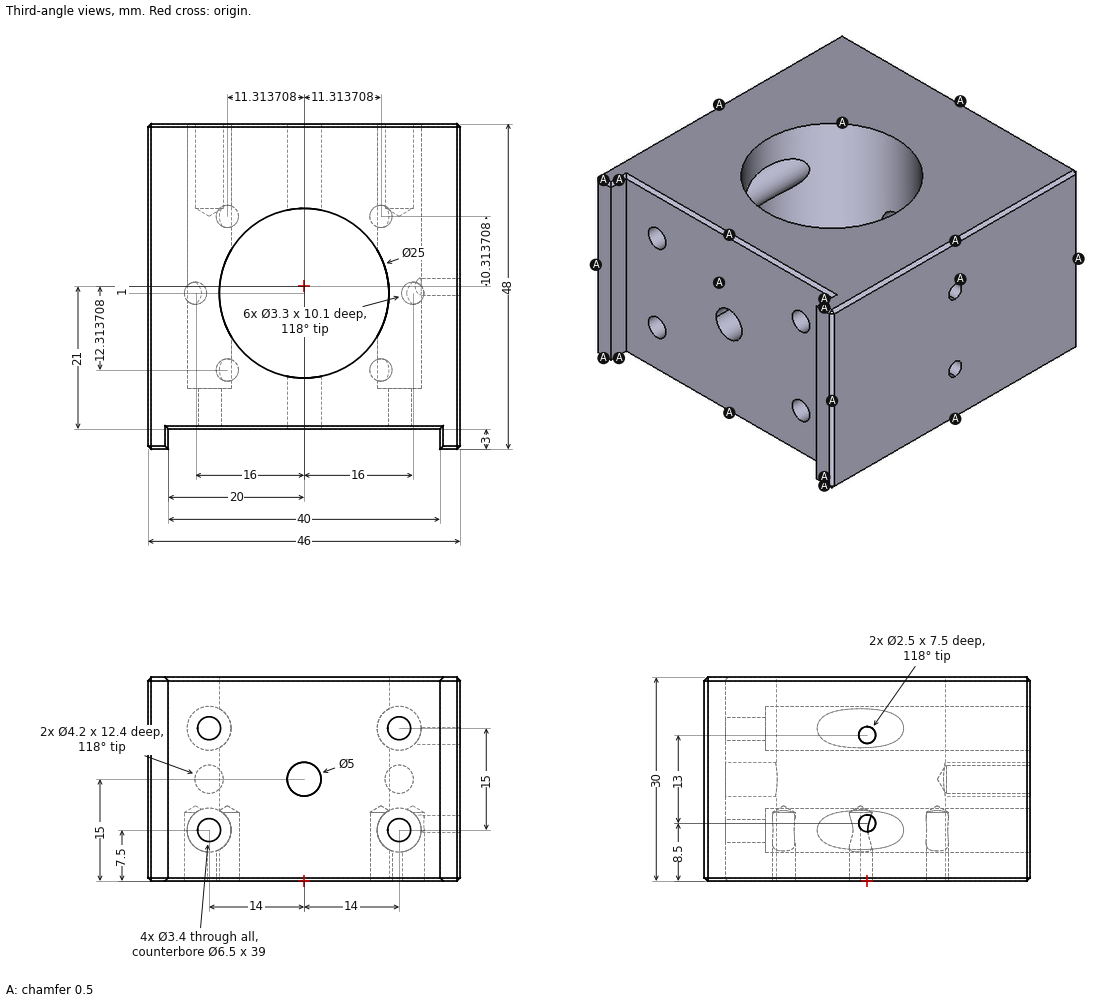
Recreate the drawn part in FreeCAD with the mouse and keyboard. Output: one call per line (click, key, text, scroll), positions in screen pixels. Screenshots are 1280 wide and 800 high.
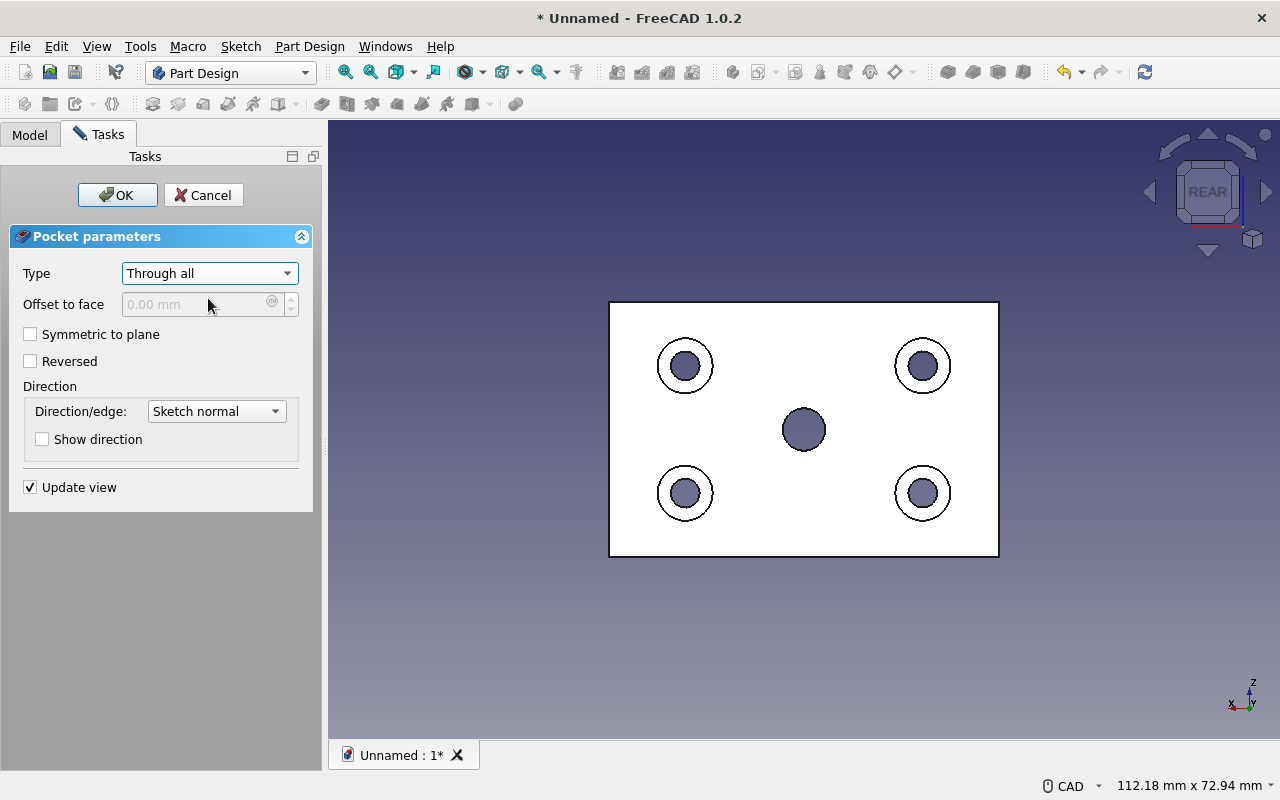
click(118, 195)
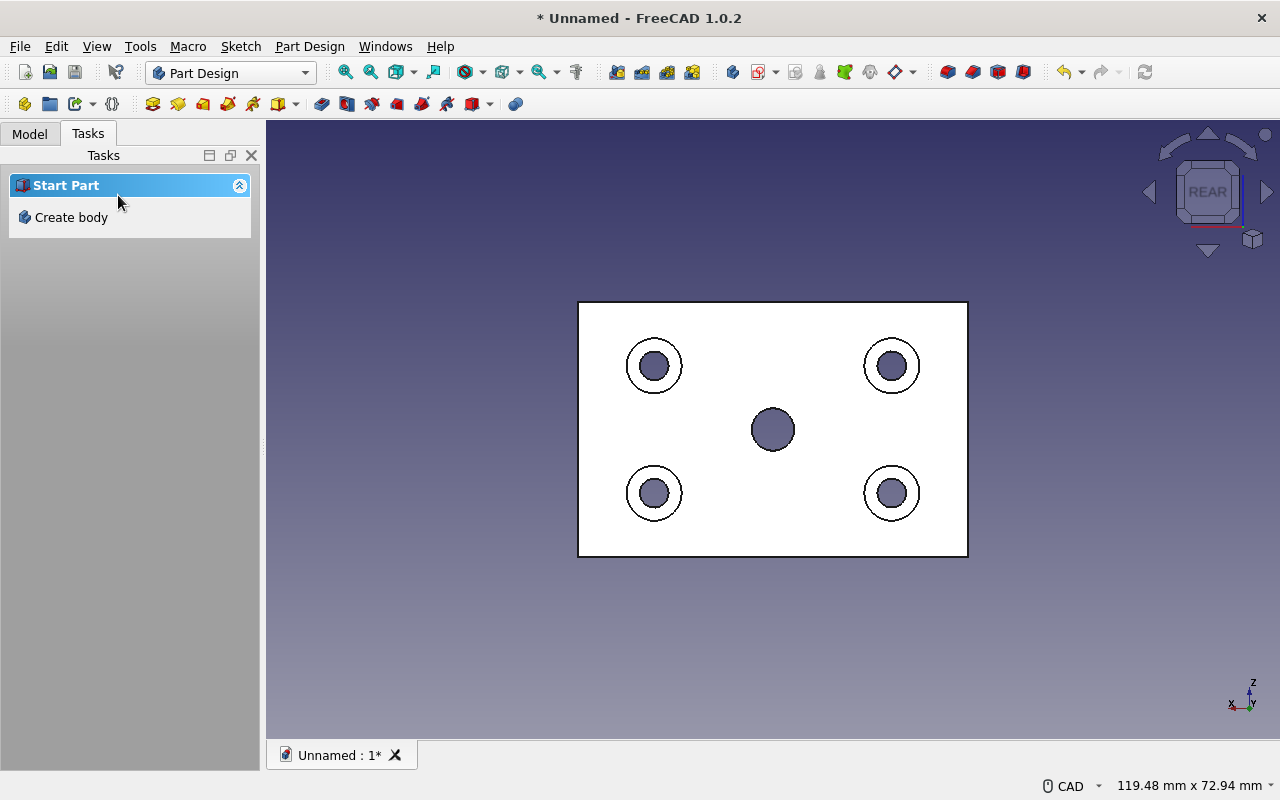
click(346, 72)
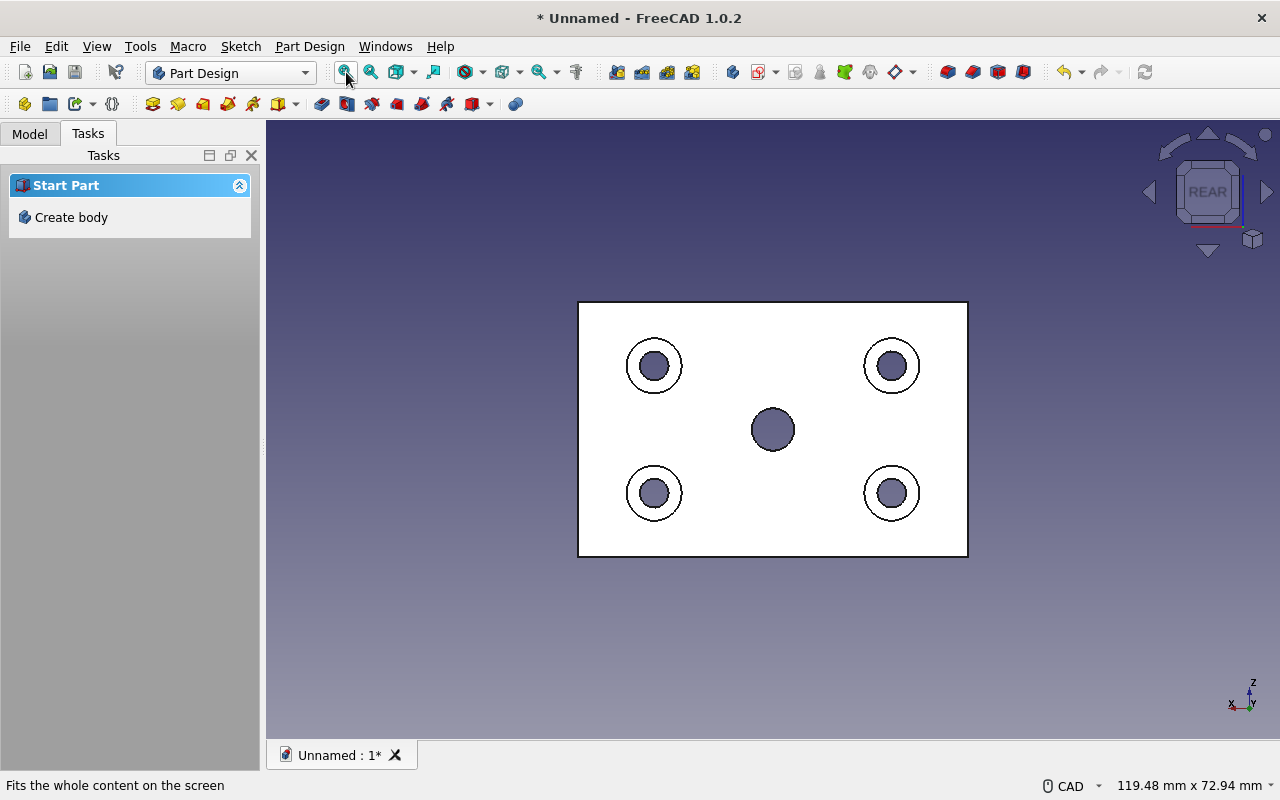
click(773, 556)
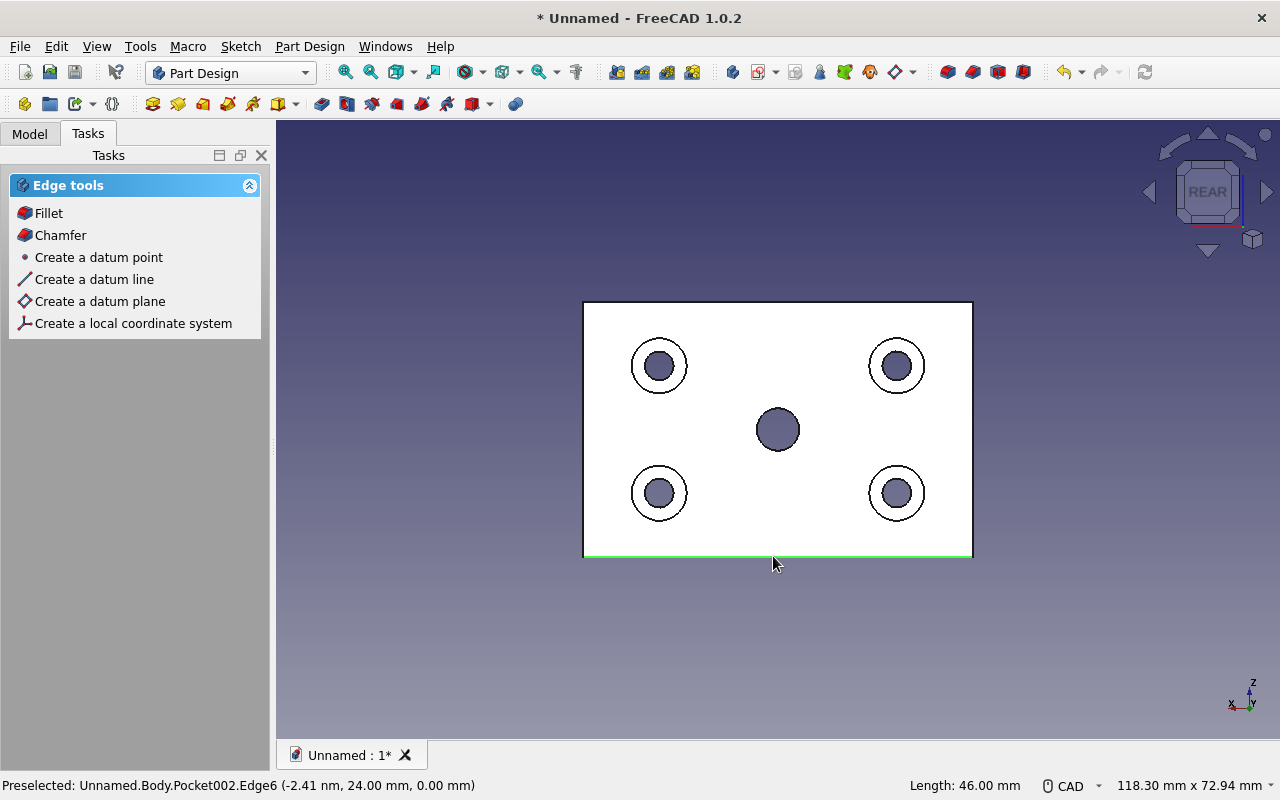
click(778, 301, ctrl)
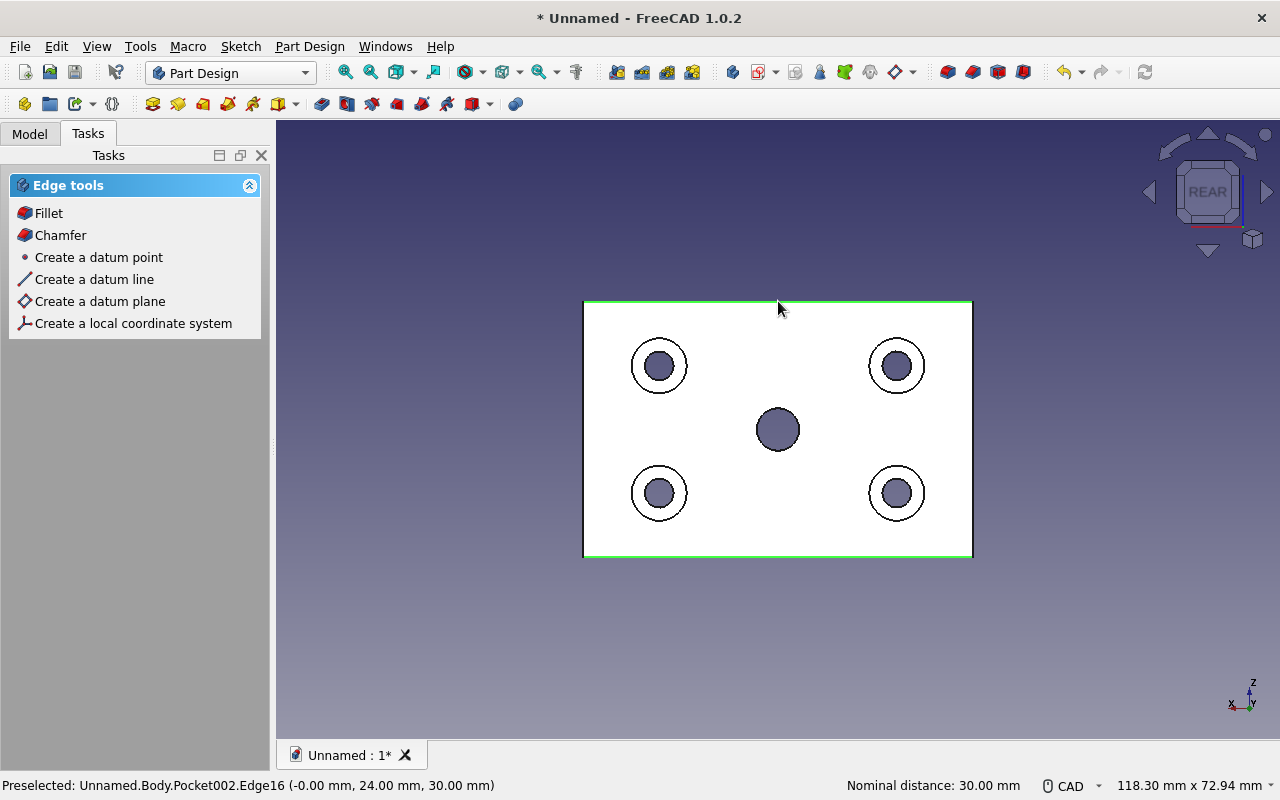
key(0)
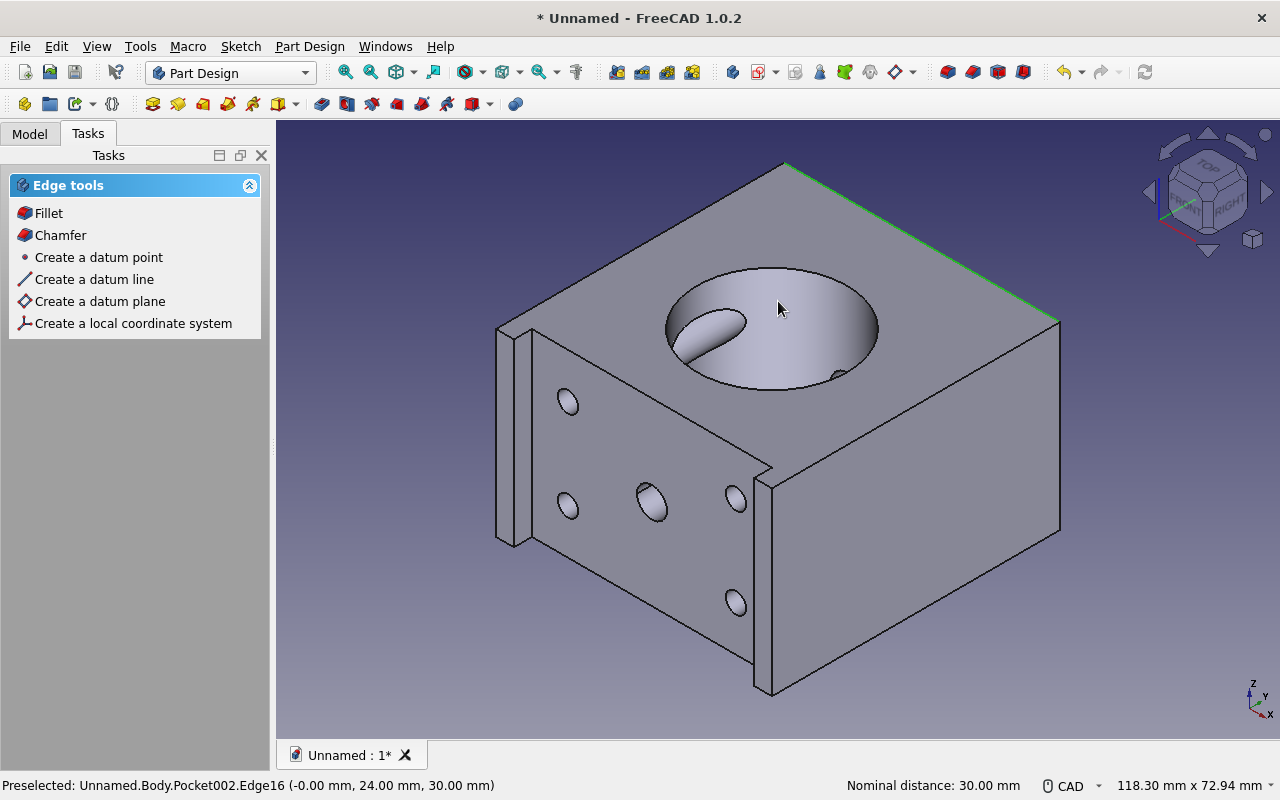
click(957, 484, ctrl)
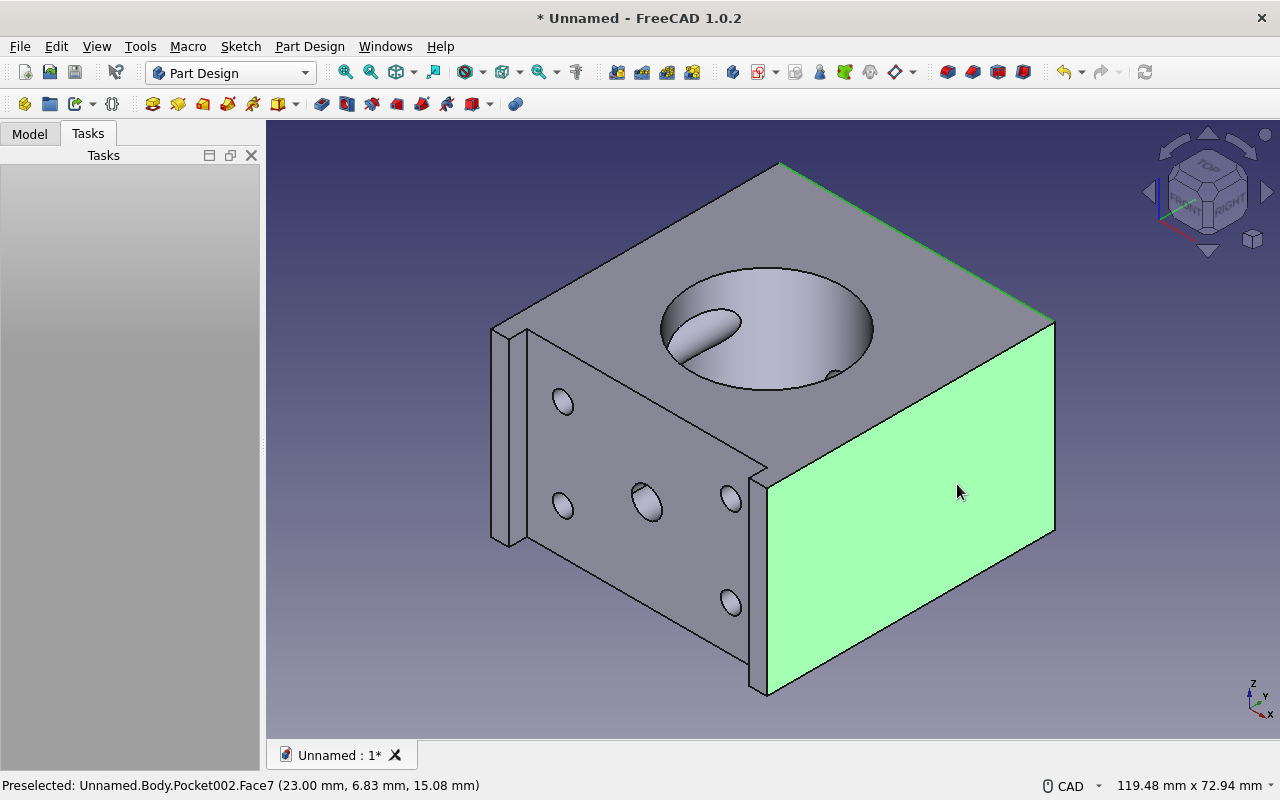
click(500, 333, ctrl)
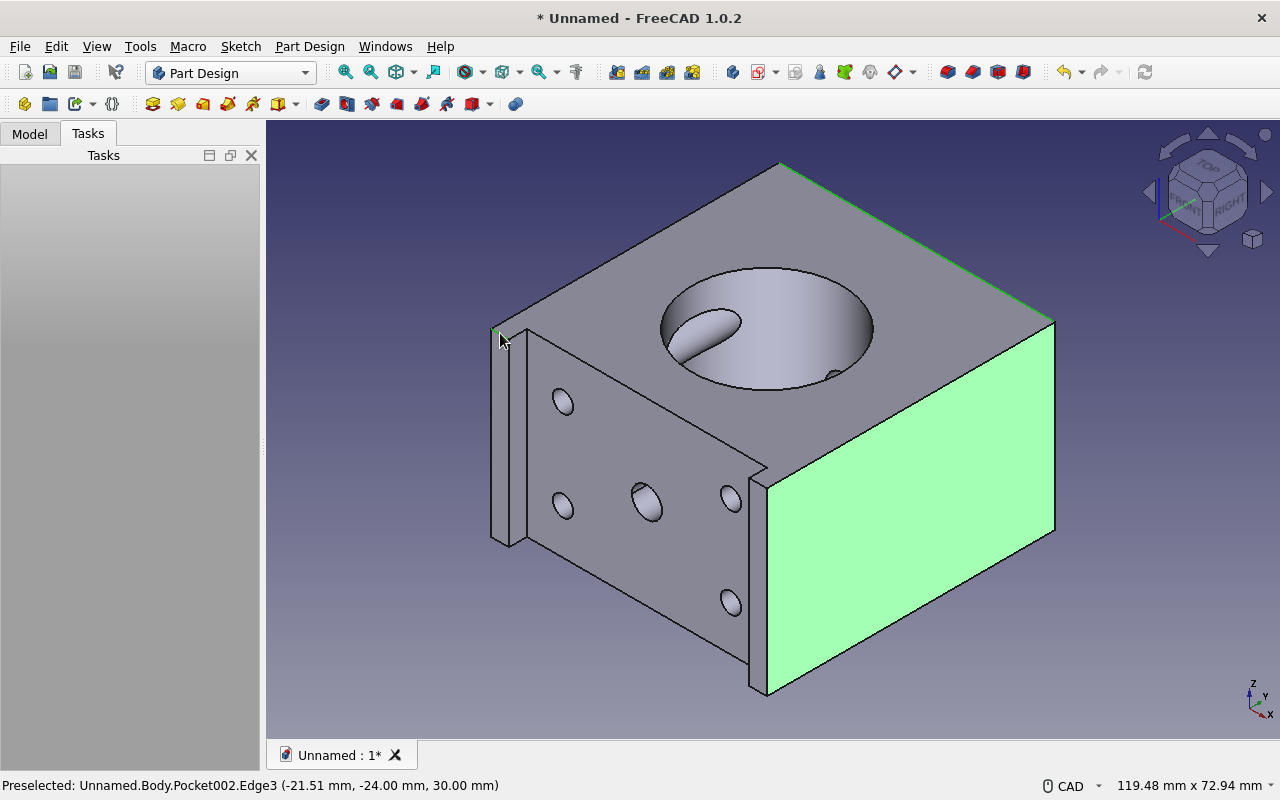
click(758, 482, ctrl)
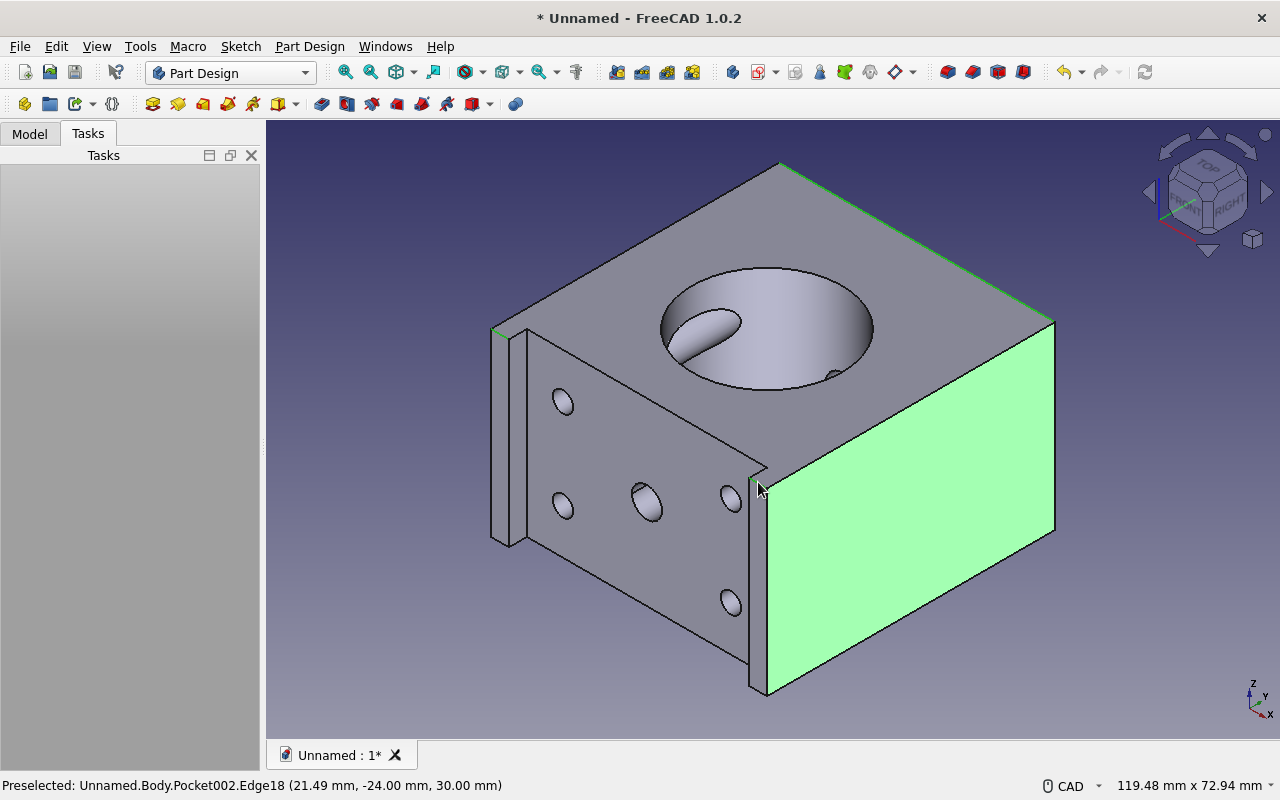
click(518, 333, ctrl)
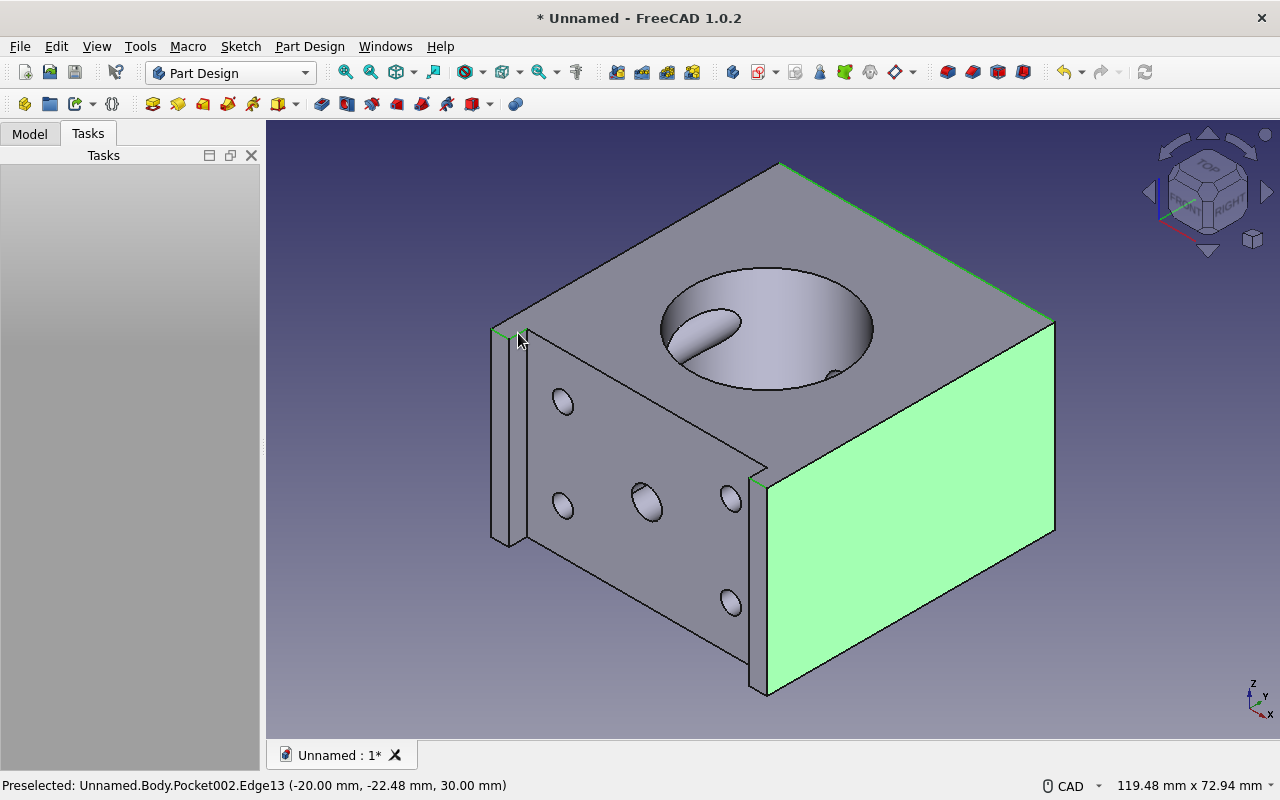
click(647, 397, ctrl)